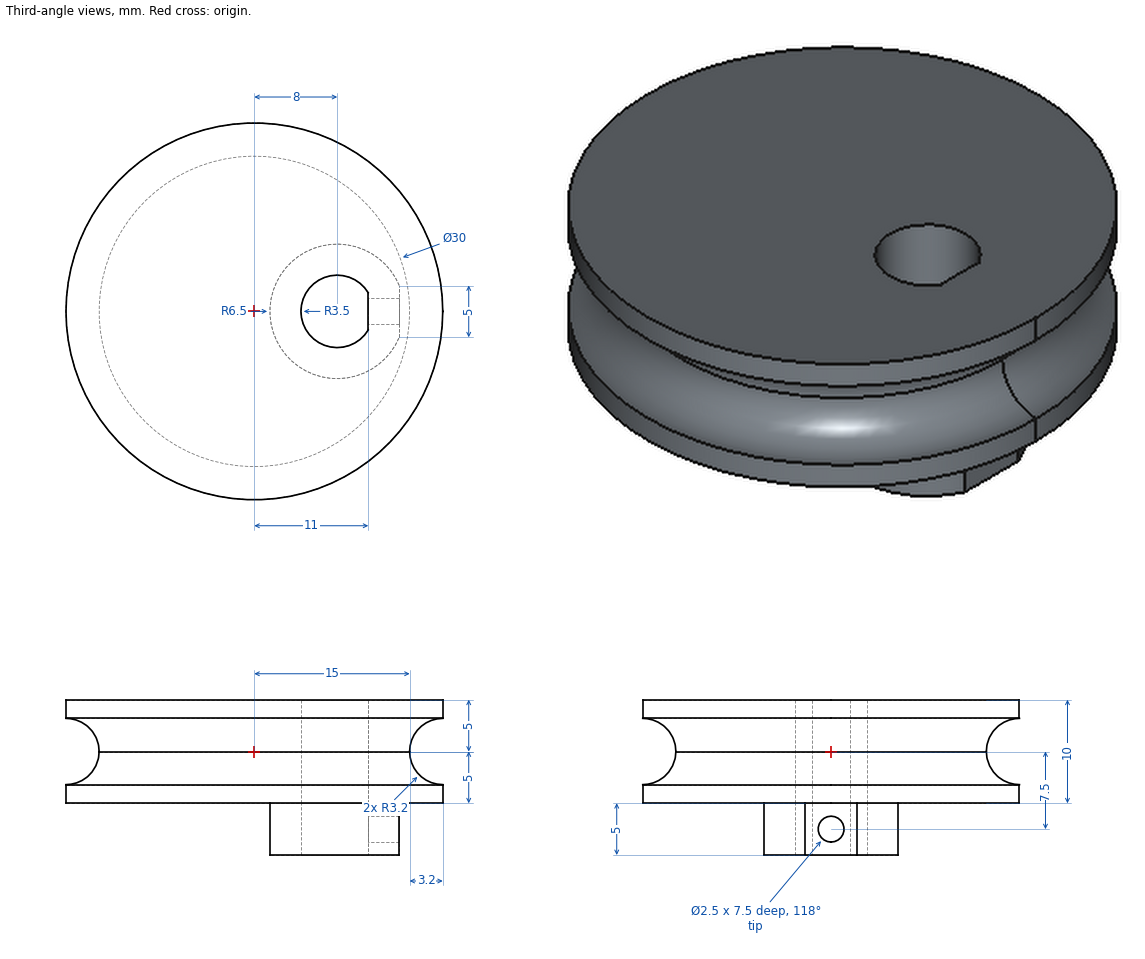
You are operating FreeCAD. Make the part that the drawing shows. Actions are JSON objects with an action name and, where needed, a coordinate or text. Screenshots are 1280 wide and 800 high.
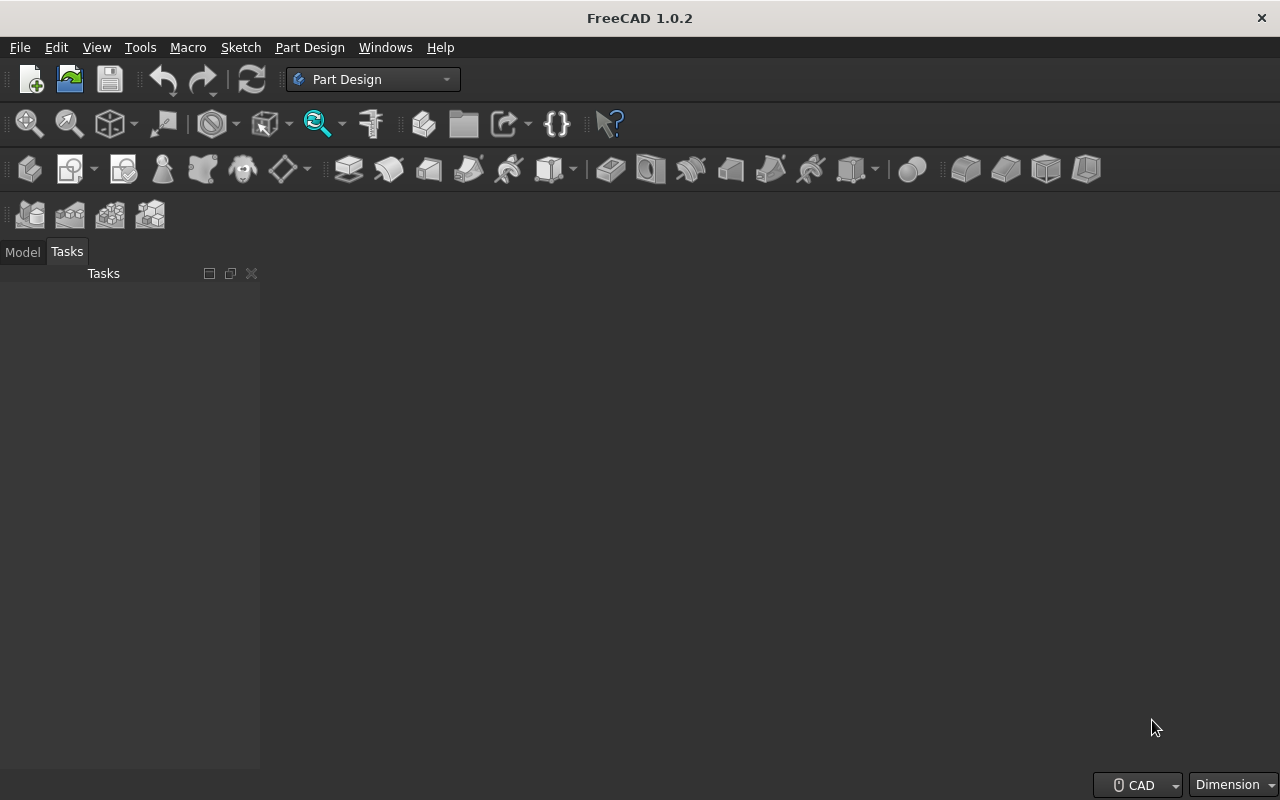
{"action": "left_click", "coordinate": [30, 80]}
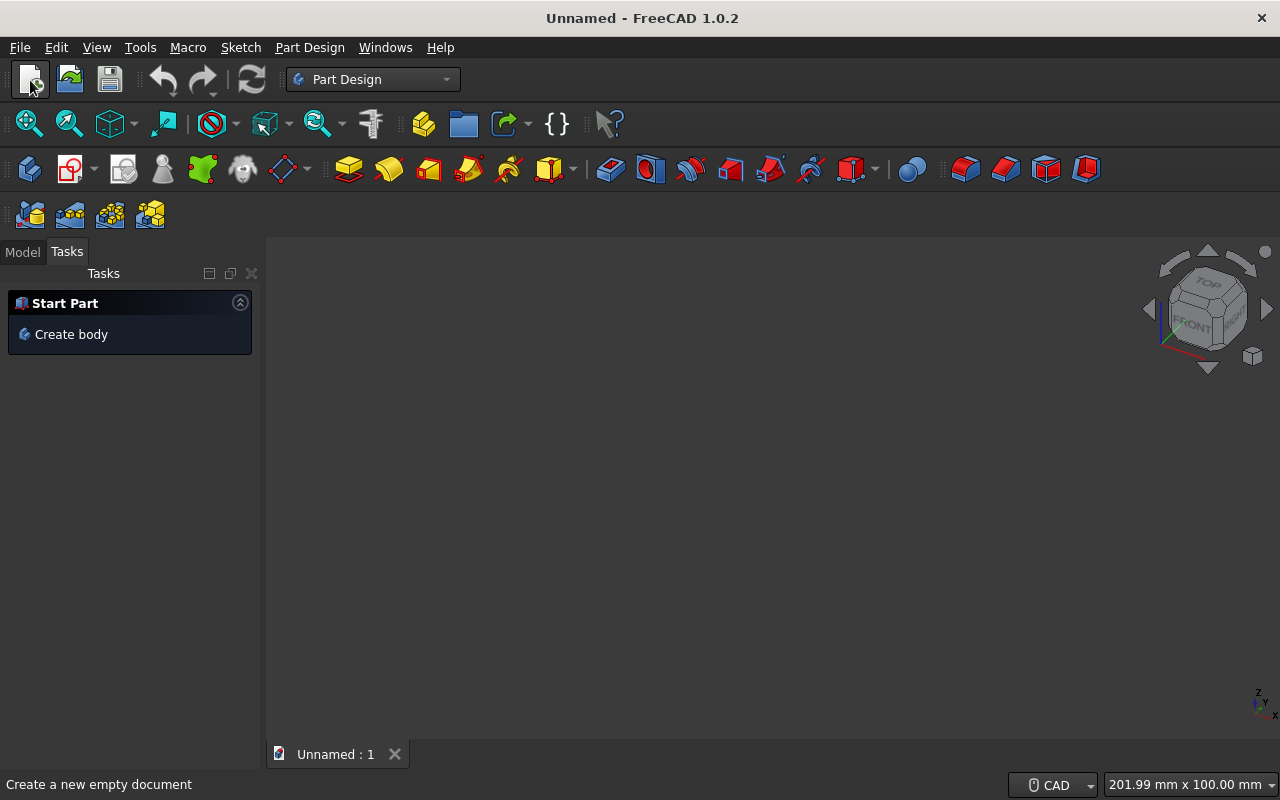
{"action": "left_click", "coordinate": [70, 170]}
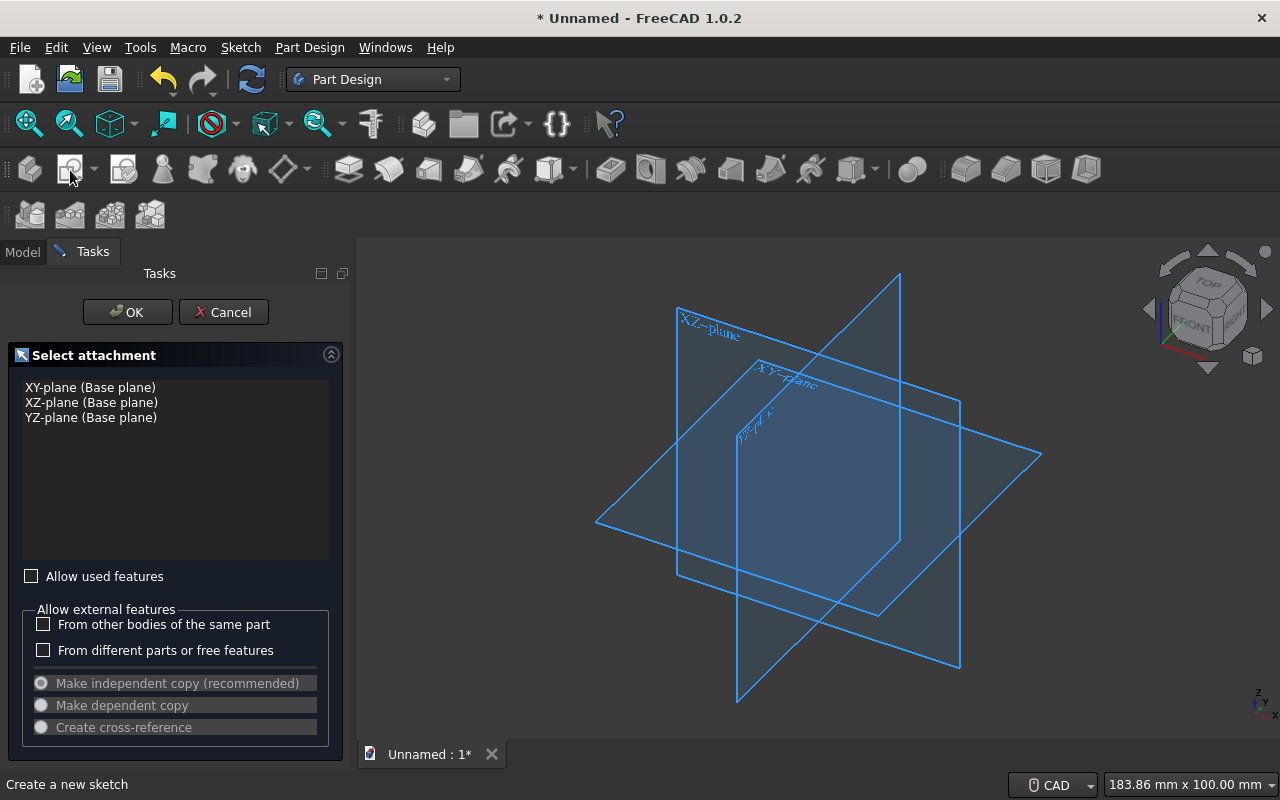
{"action": "left_click", "coordinate": [82, 388]}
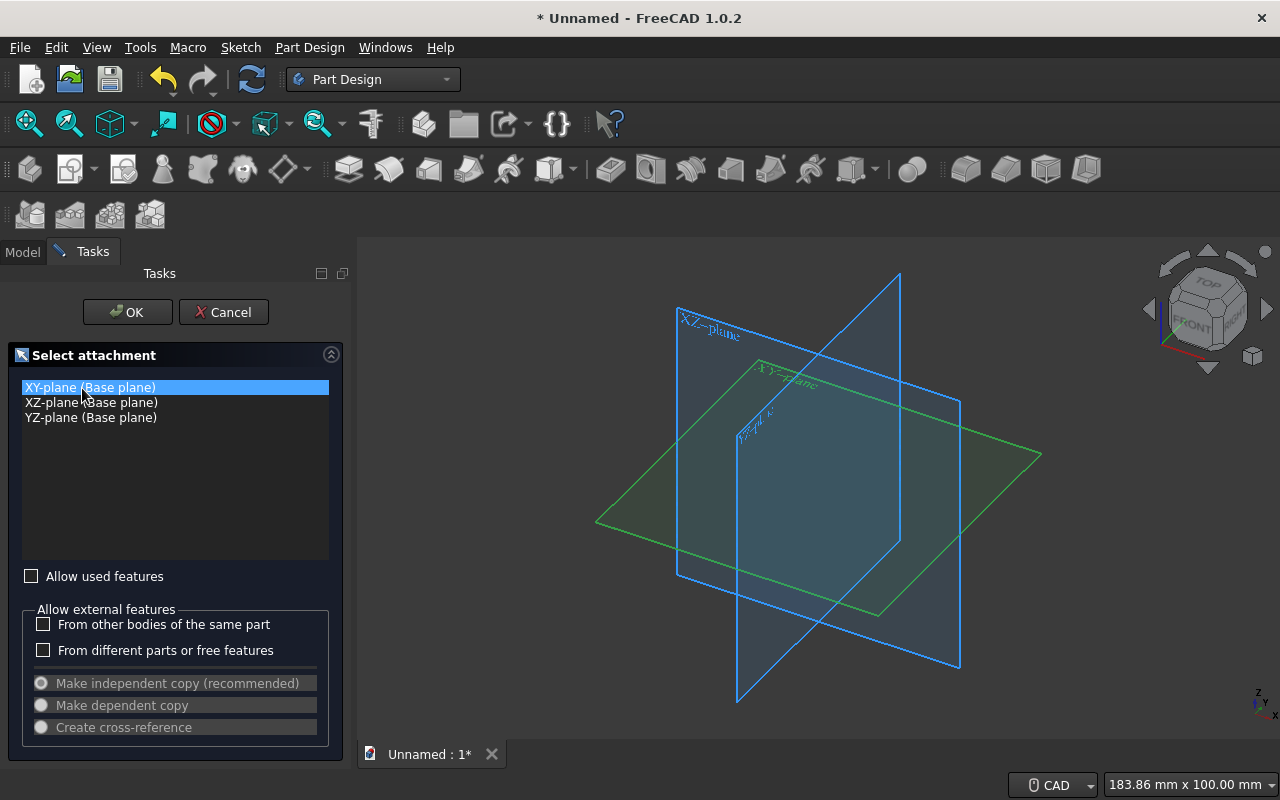
{"action": "left_click", "coordinate": [128, 312]}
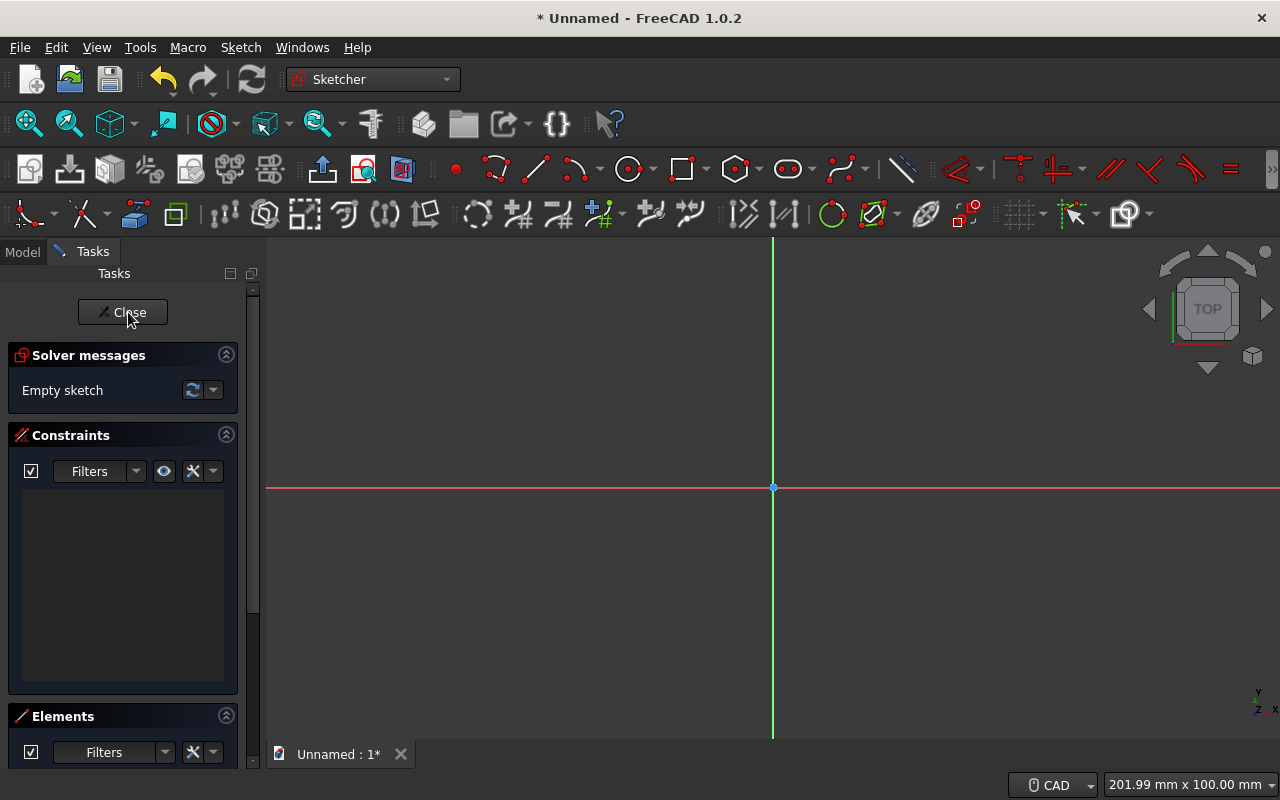
{"action": "scroll", "coordinate": [829, 488], "scroll_direction": "up", "scroll_amount": 4}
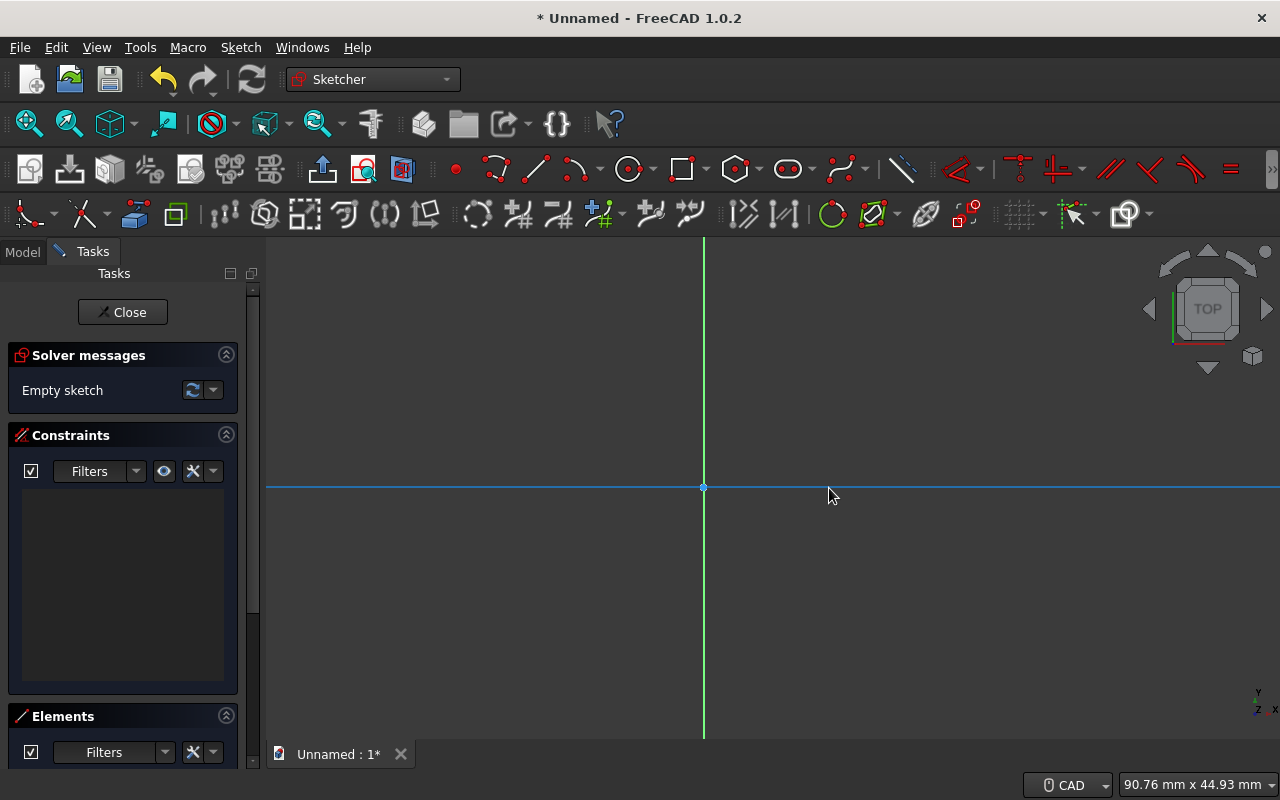
{"action": "left_click", "coordinate": [536, 170]}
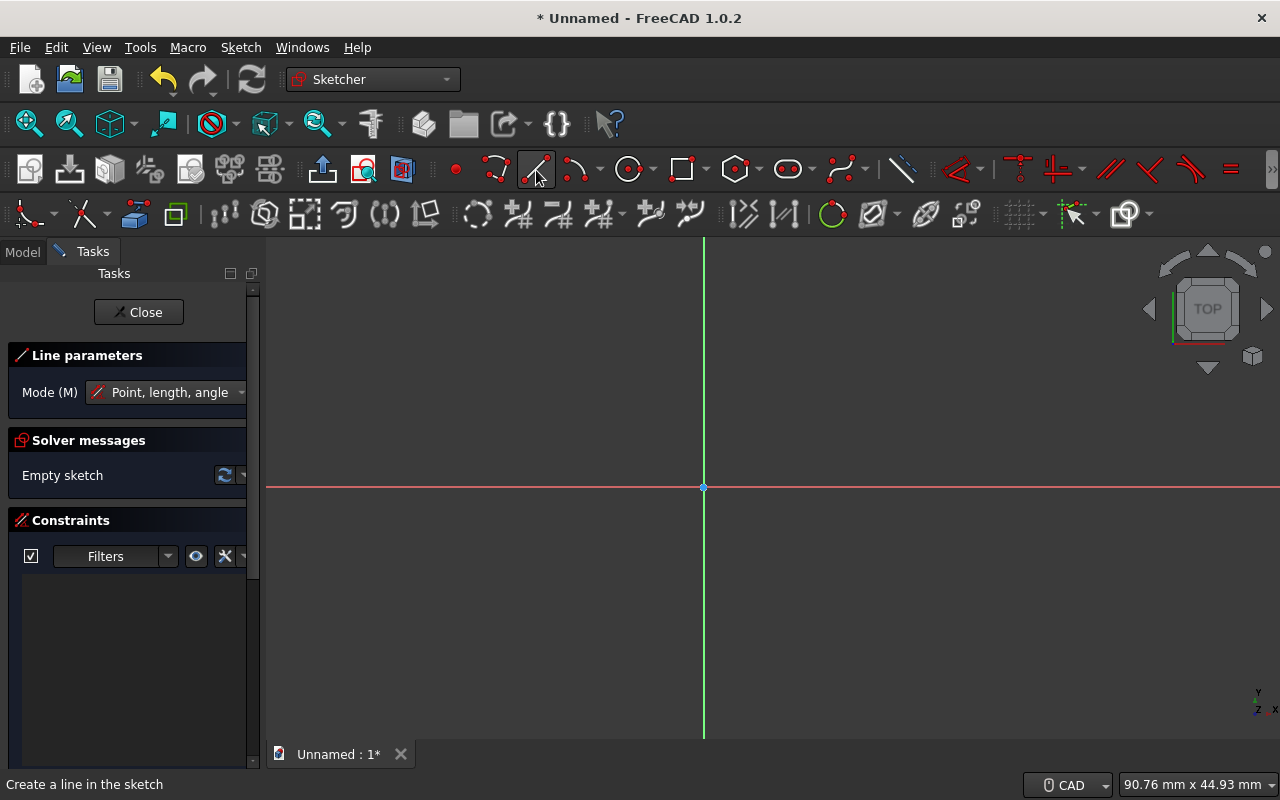
{"action": "left_click", "coordinate": [827, 508]}
{"action": "left_click", "coordinate": [827, 467]}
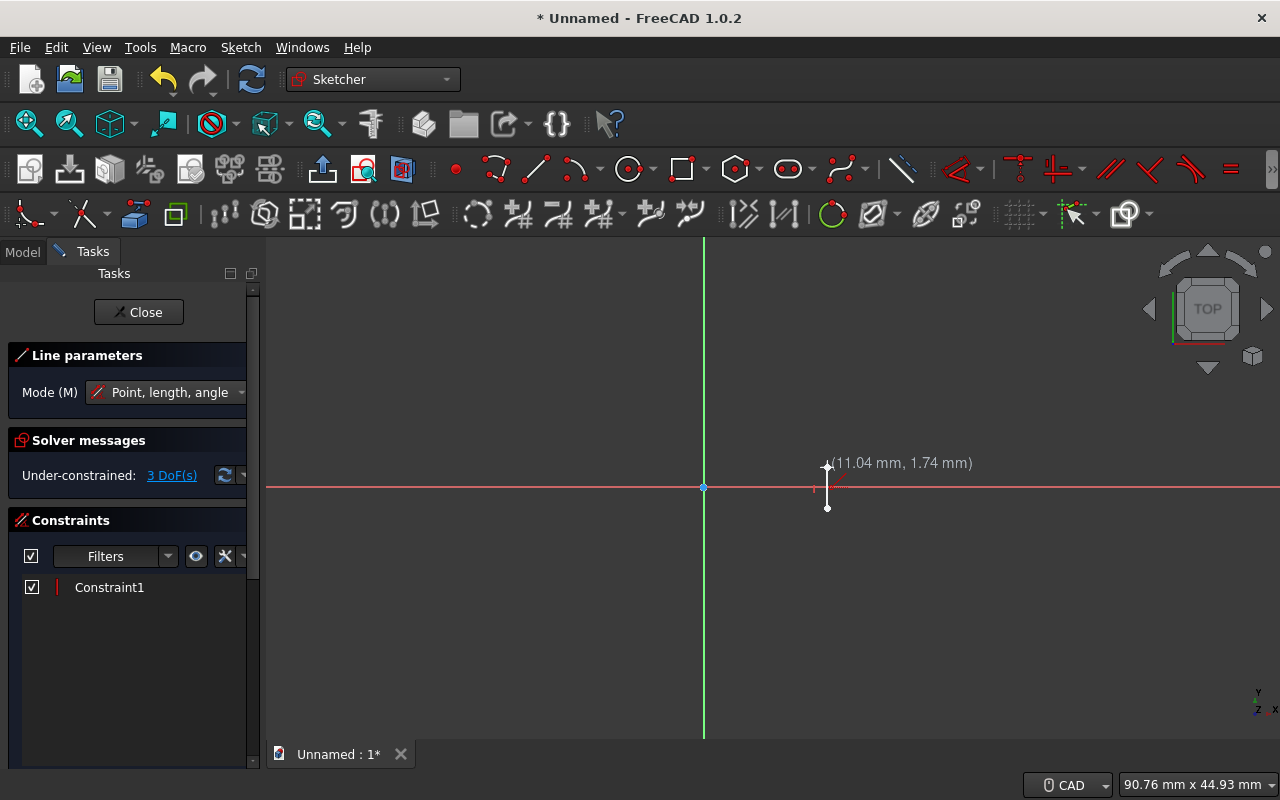
{"action": "left_click", "coordinate": [602, 170]}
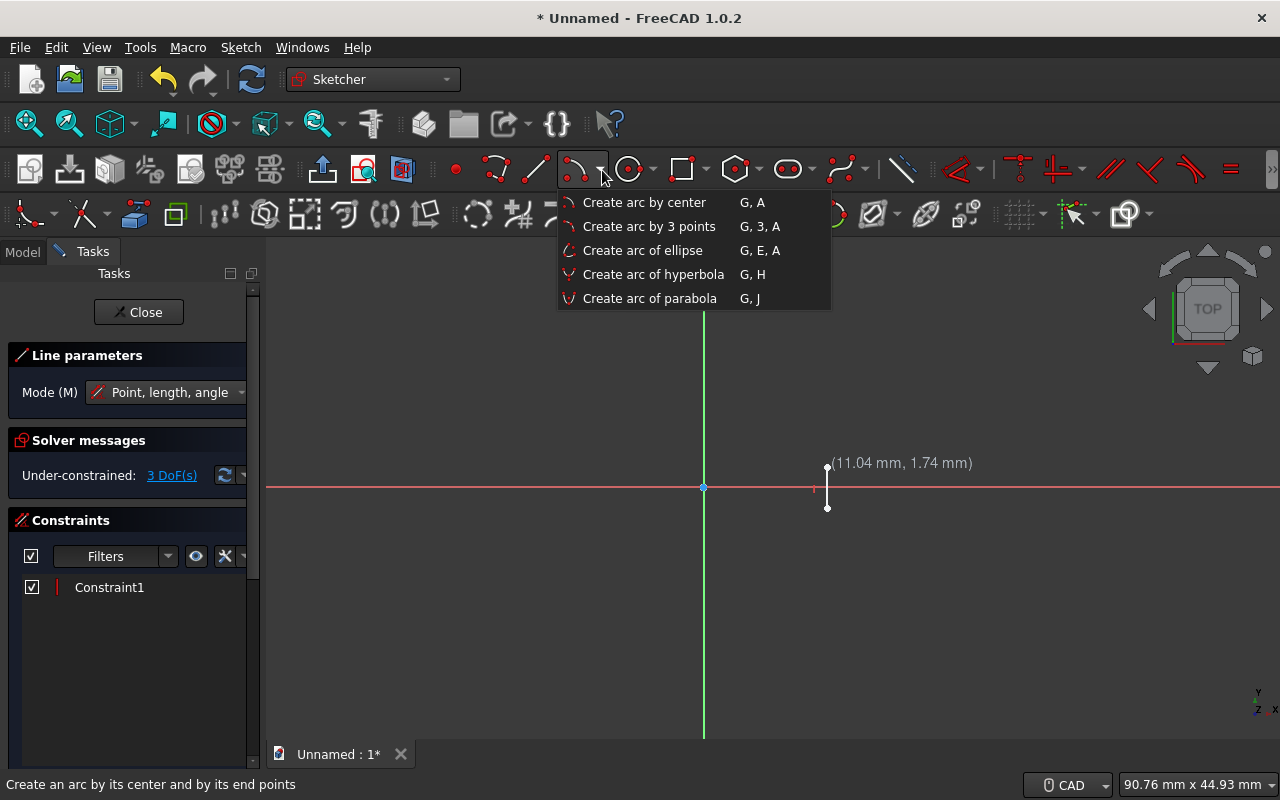
{"action": "left_click", "coordinate": [694, 226]}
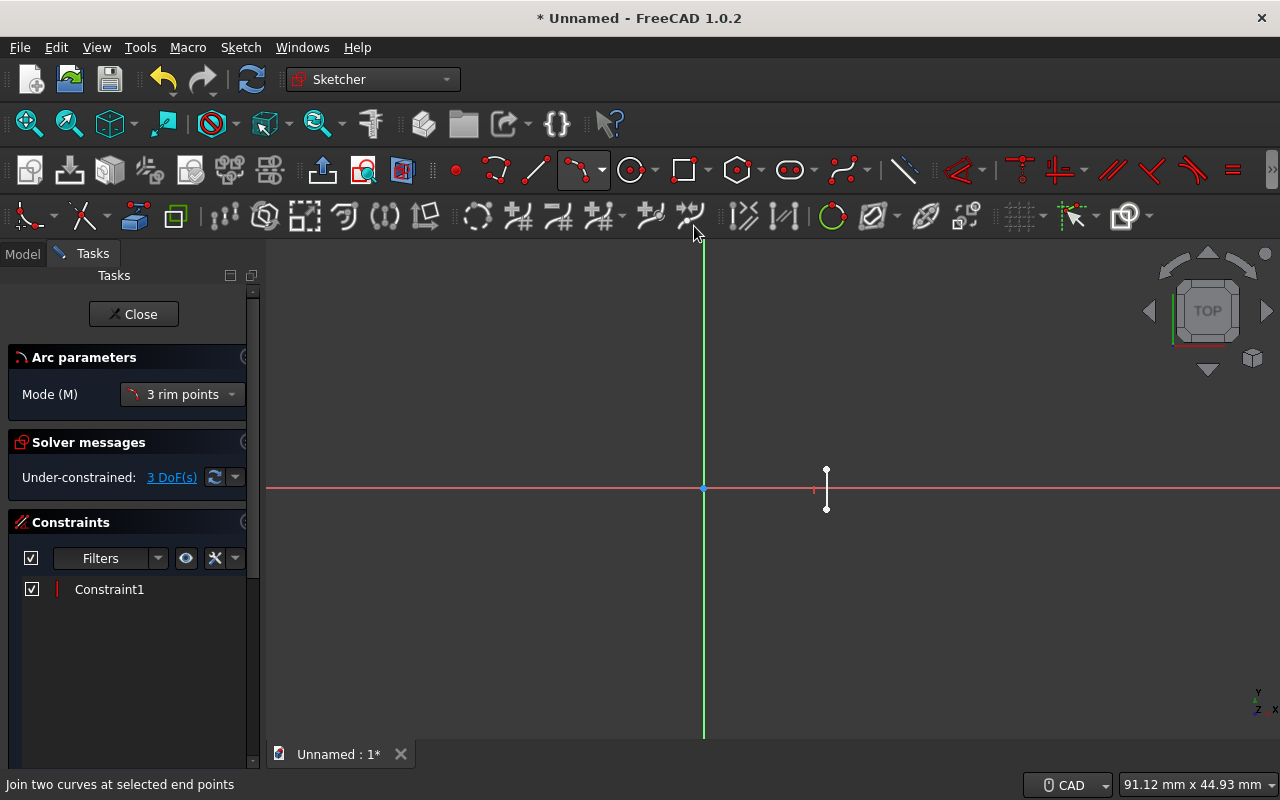
{"action": "left_click", "coordinate": [827, 469]}
{"action": "left_click", "coordinate": [827, 510]}
{"action": "left_click", "coordinate": [759, 469]}